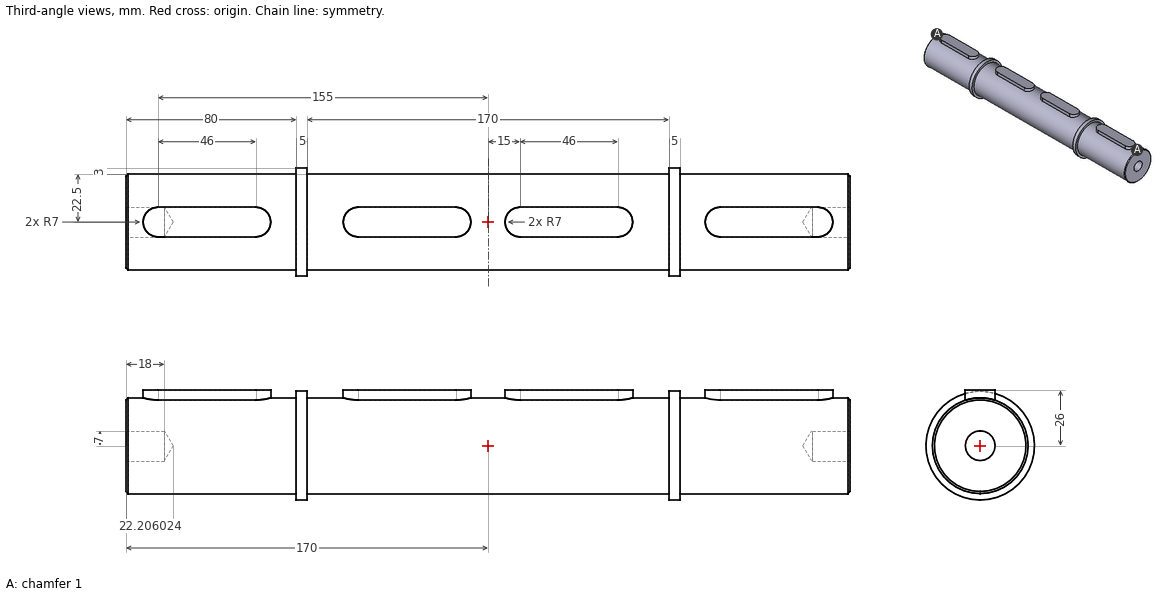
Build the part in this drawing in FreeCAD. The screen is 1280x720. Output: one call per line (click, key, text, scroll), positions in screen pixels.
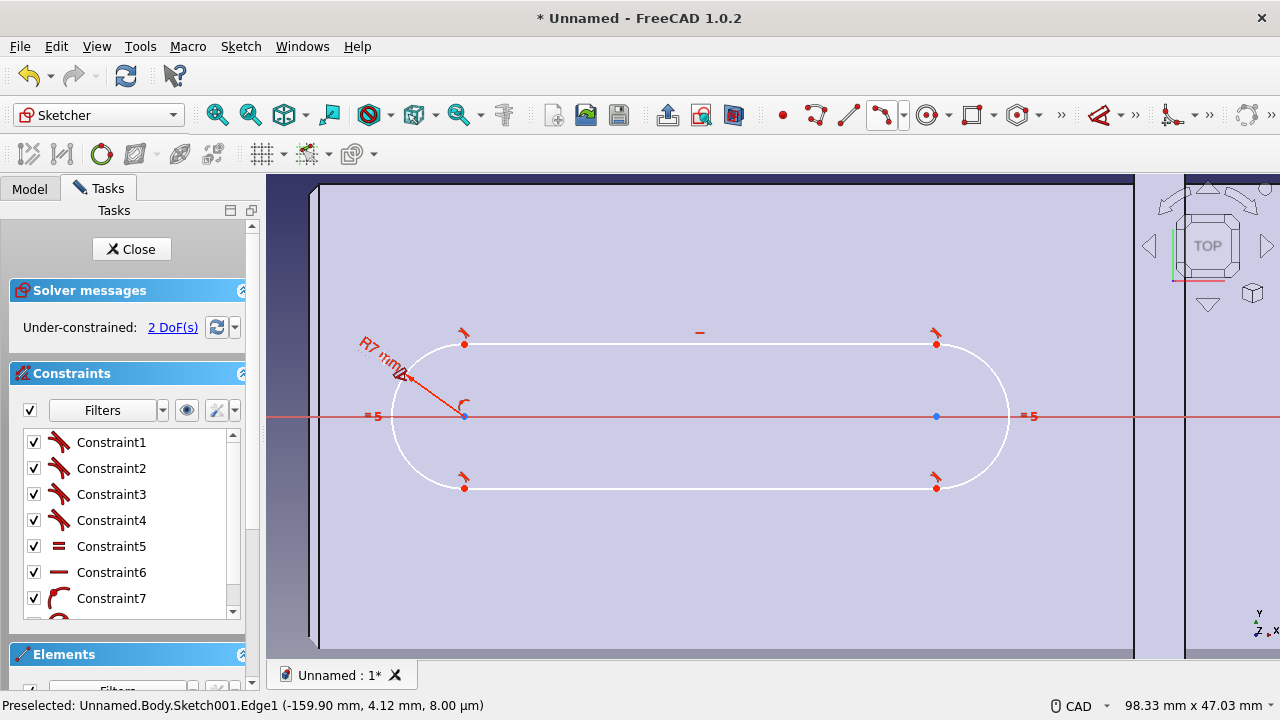
click(606, 344)
click(700, 310)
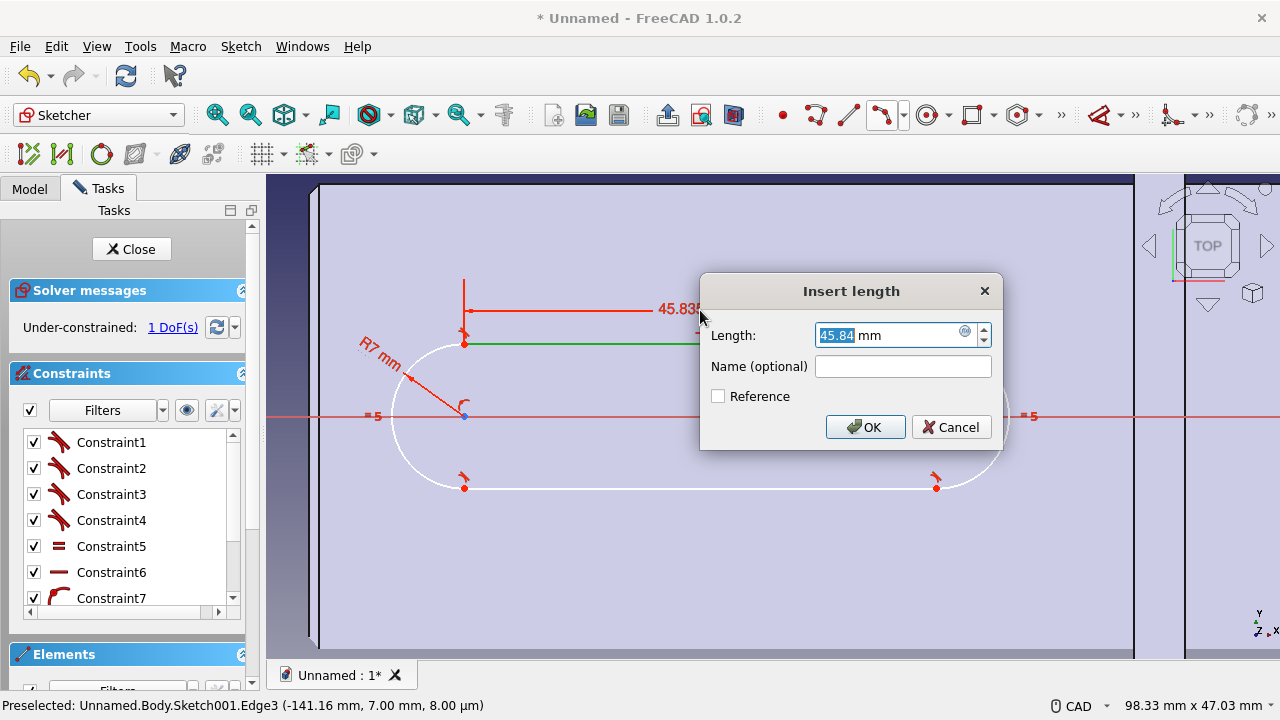
text(46)
key(Return)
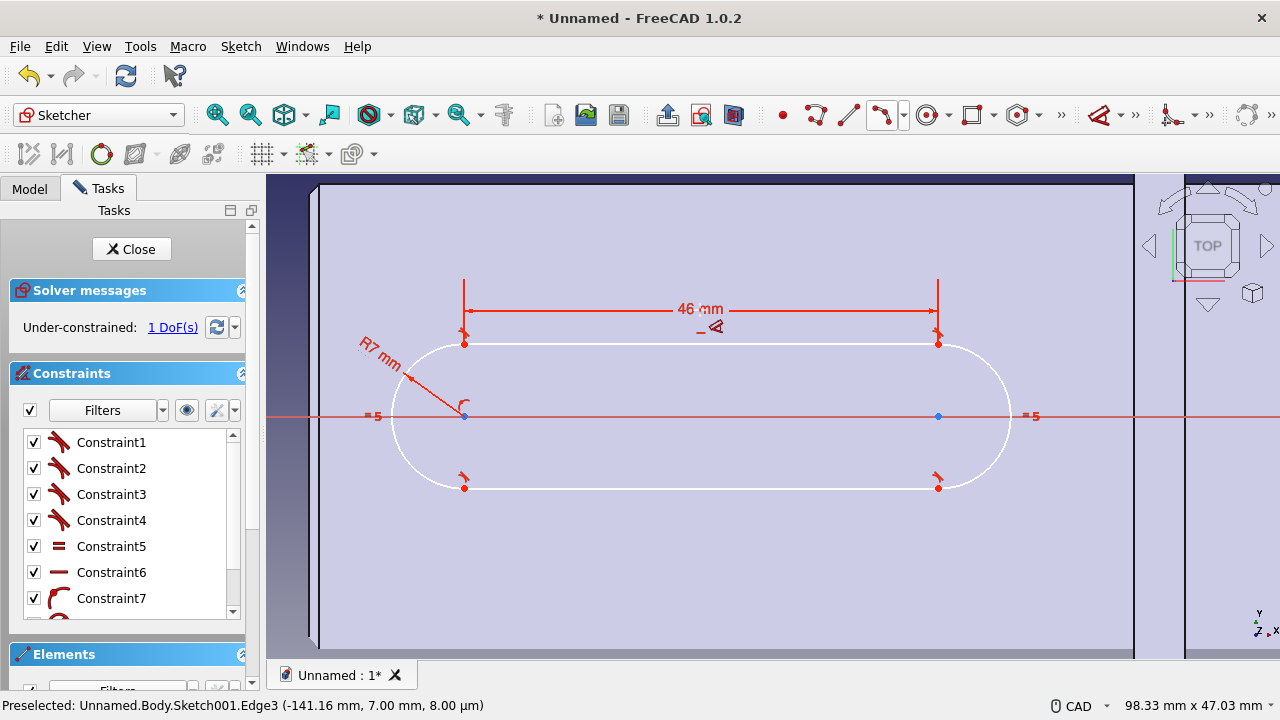
click(464, 344)
click(790, 310)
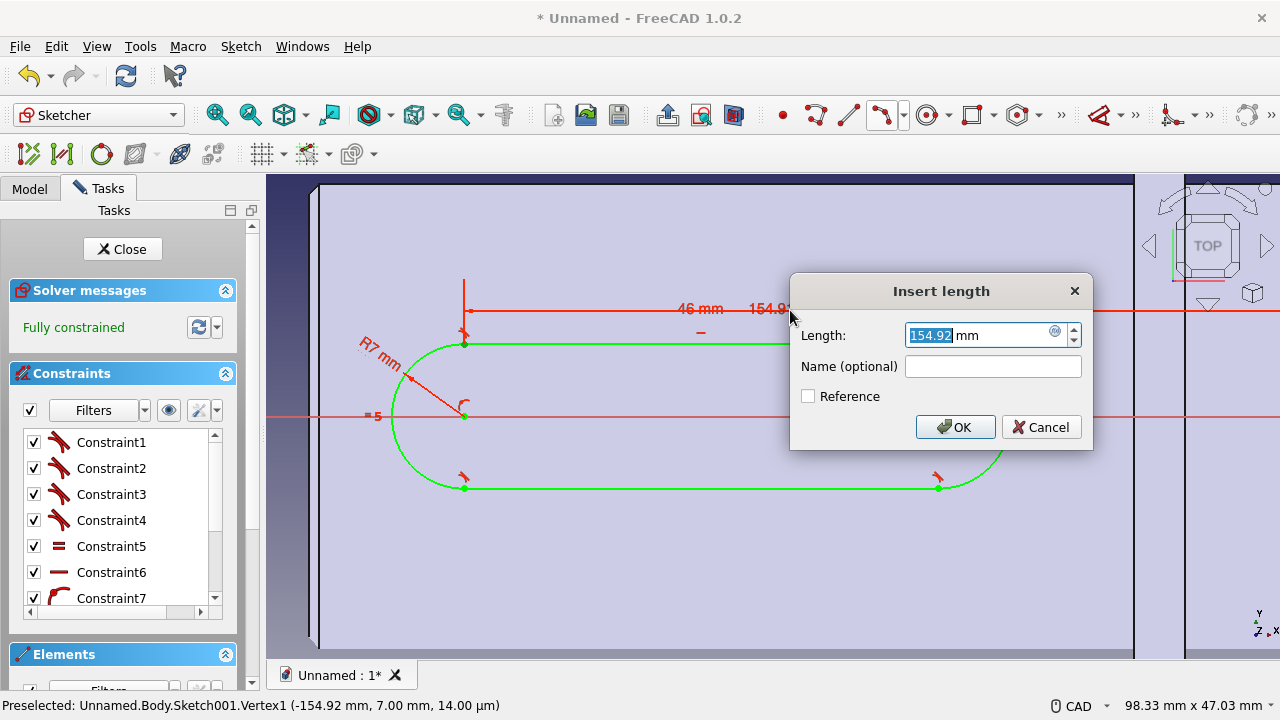
text(155)
key(Return)
key(Escape)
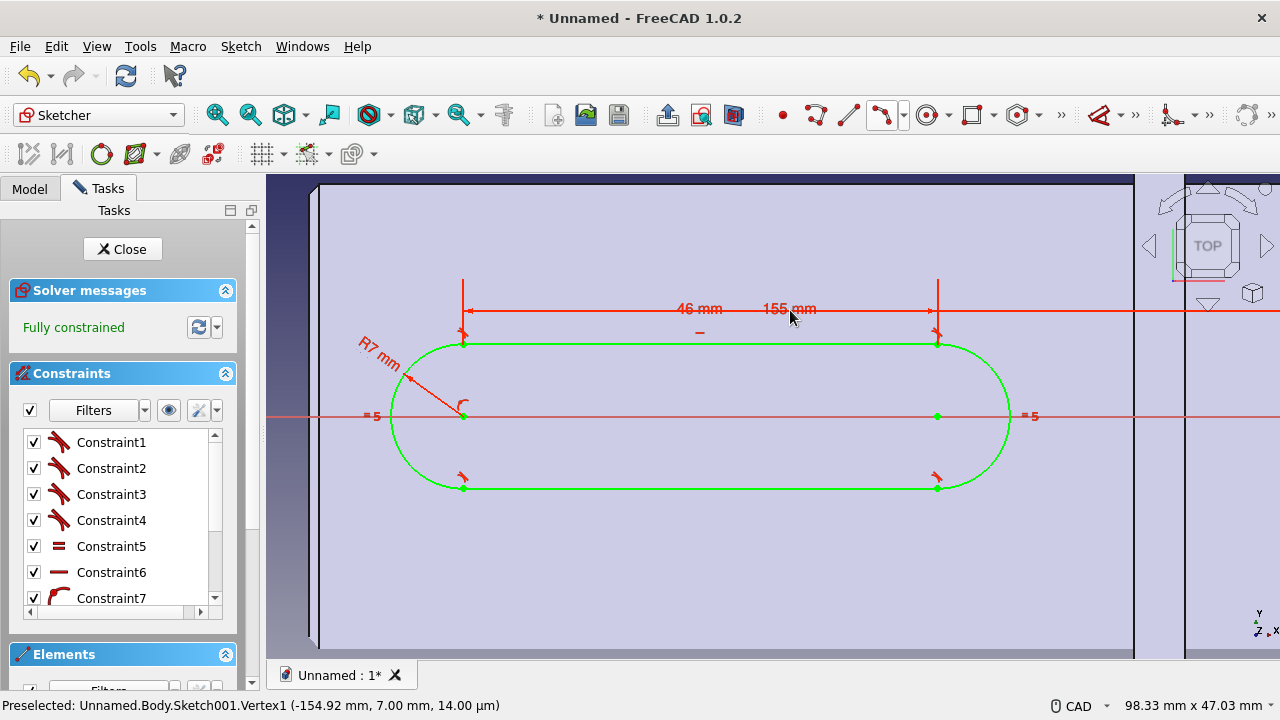
click(123, 249)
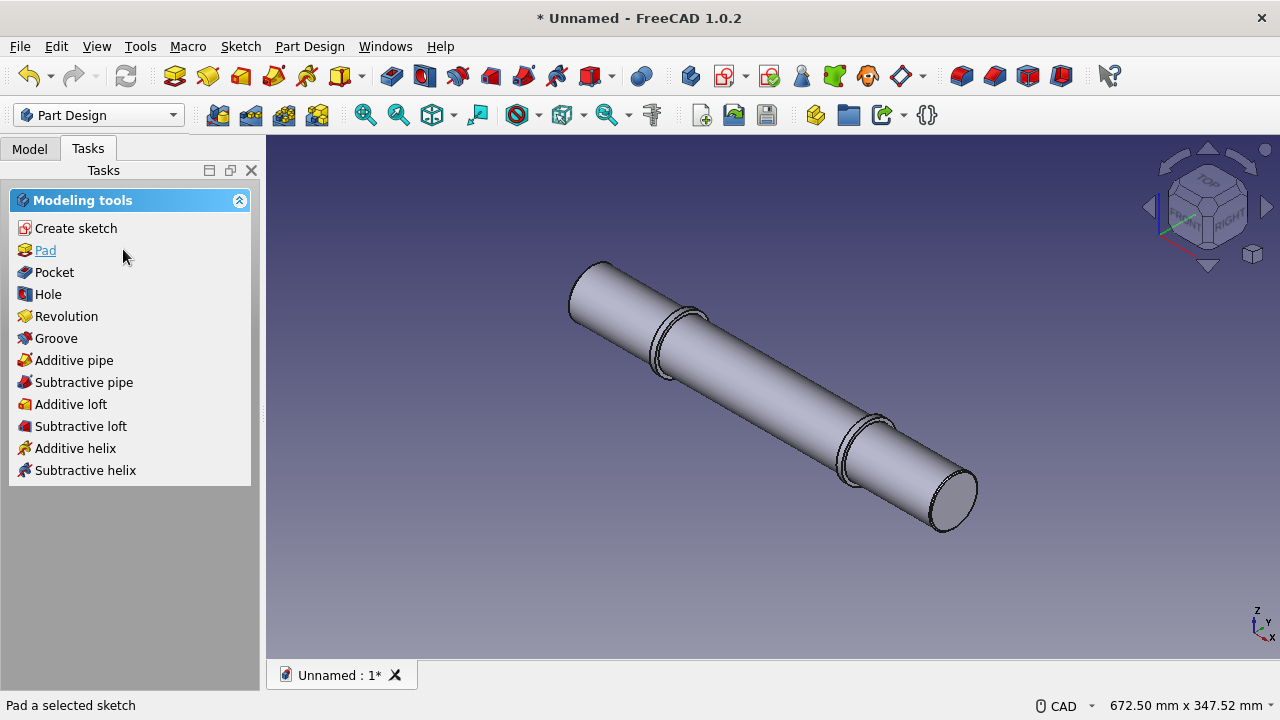
click(175, 76)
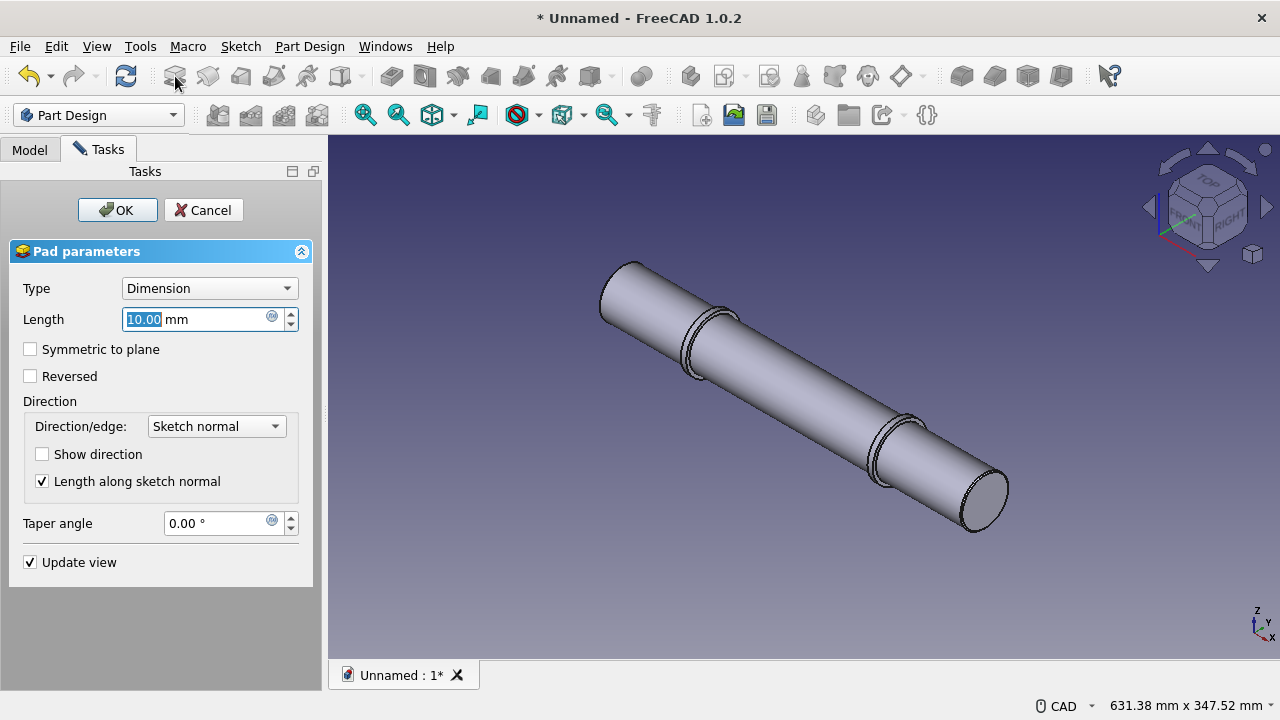
text(26)
key(Tab)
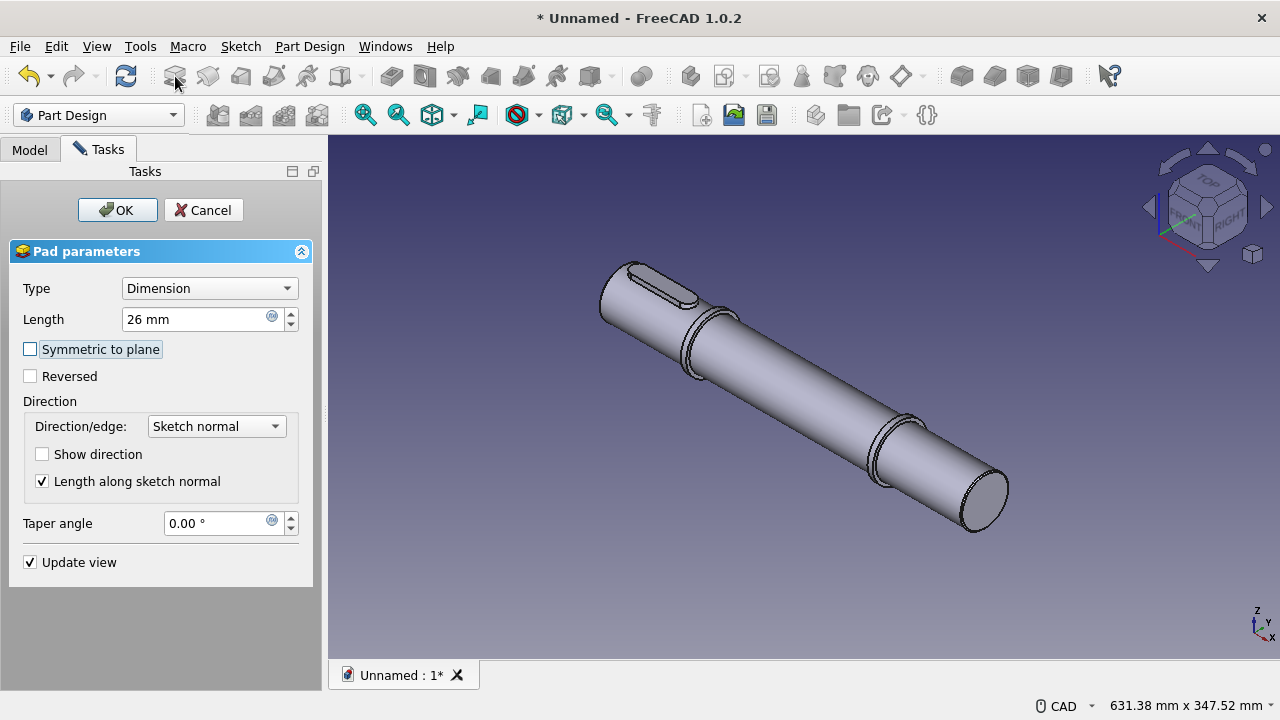
click(118, 210)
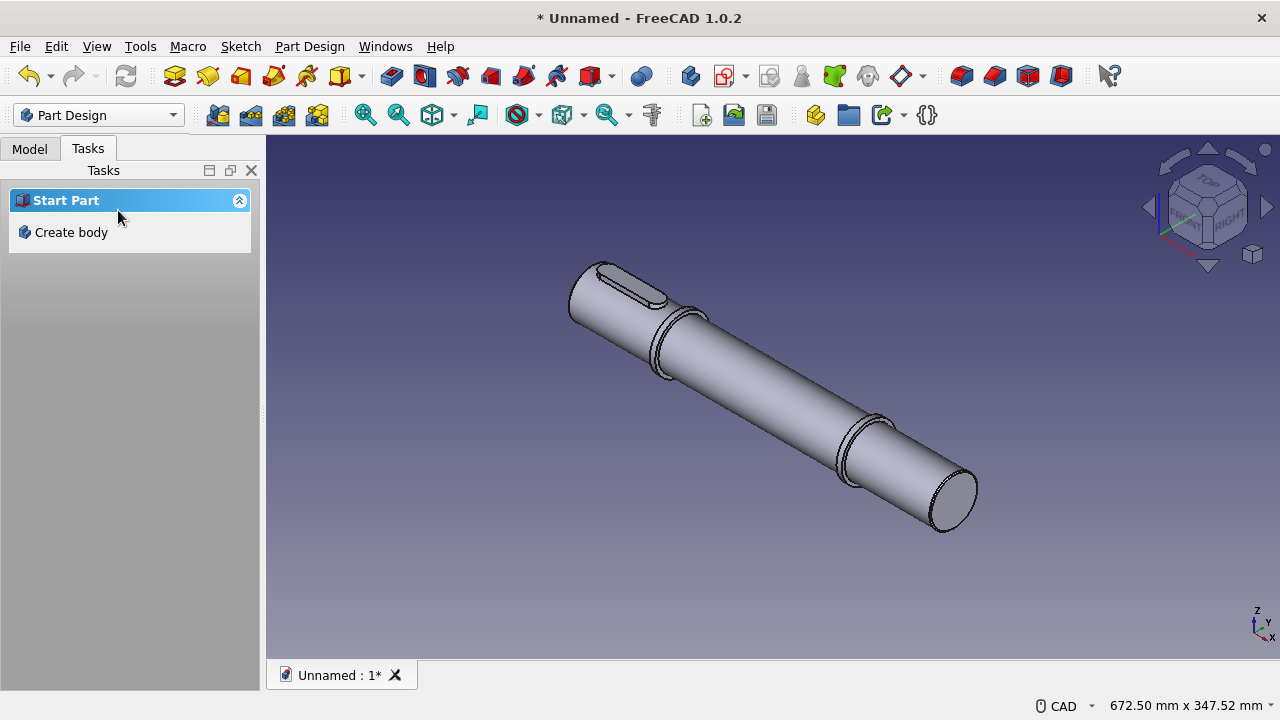
click(30, 148)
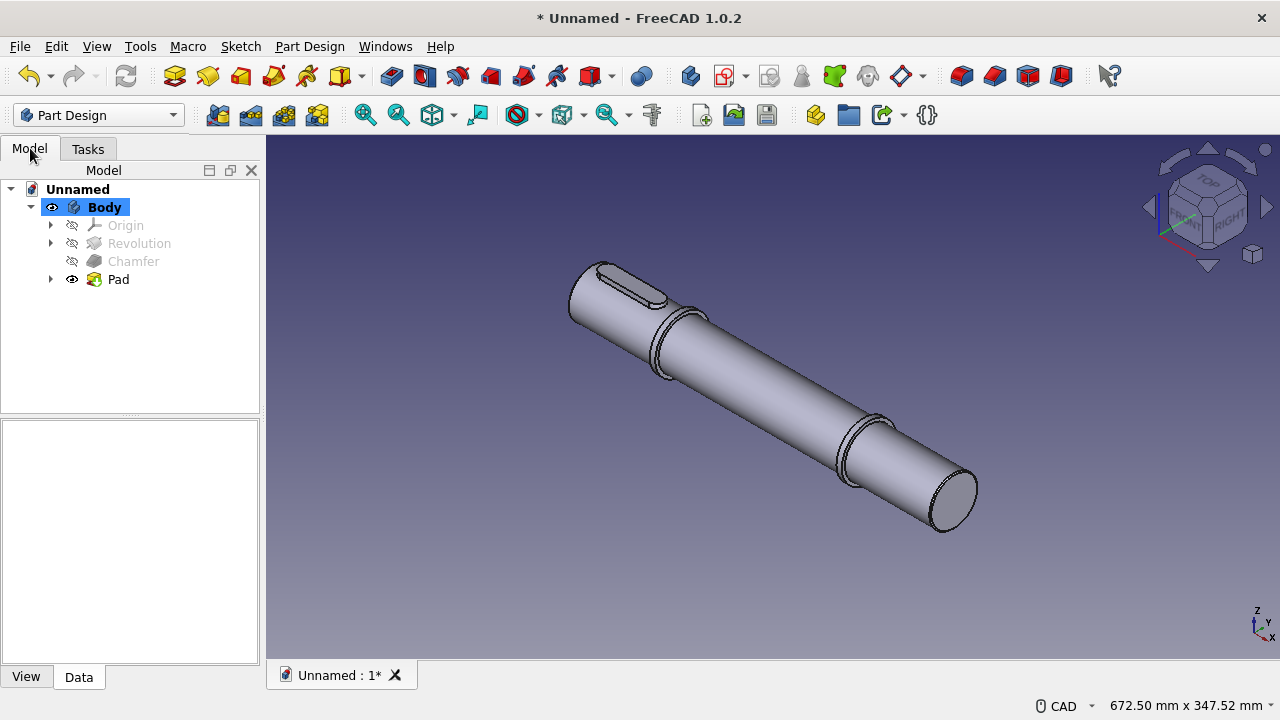
click(117, 279)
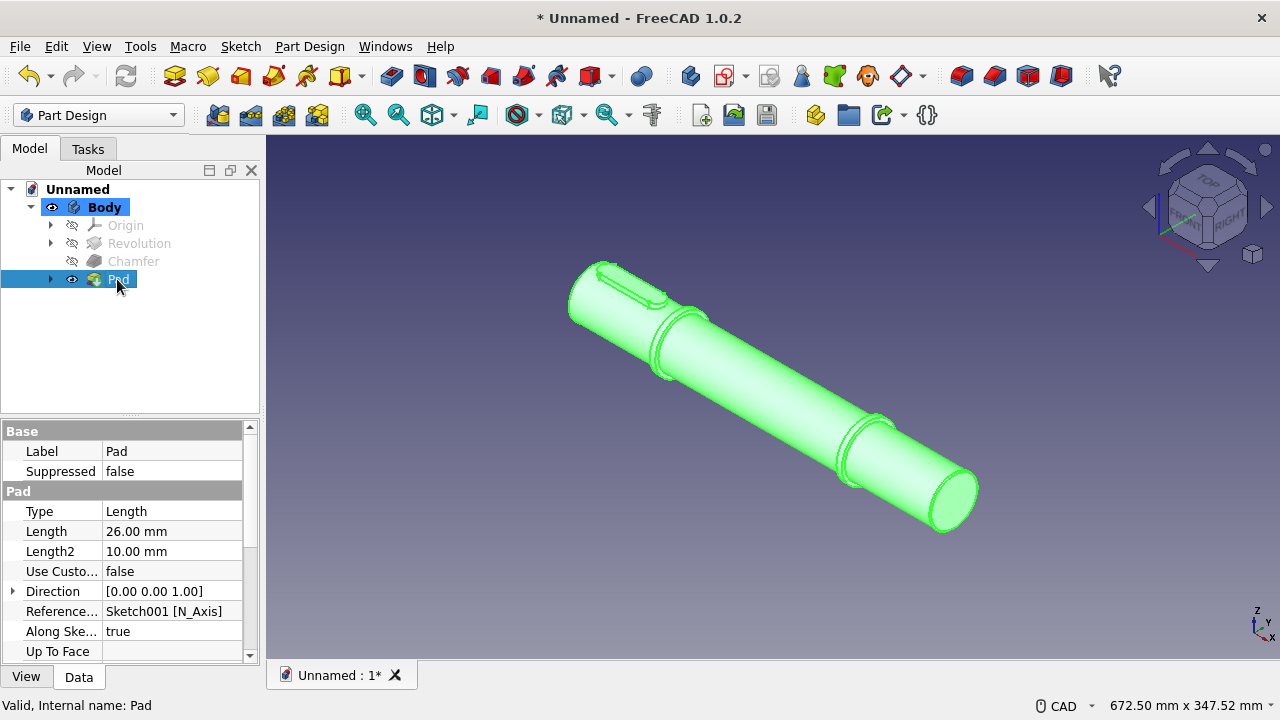
click(218, 116)